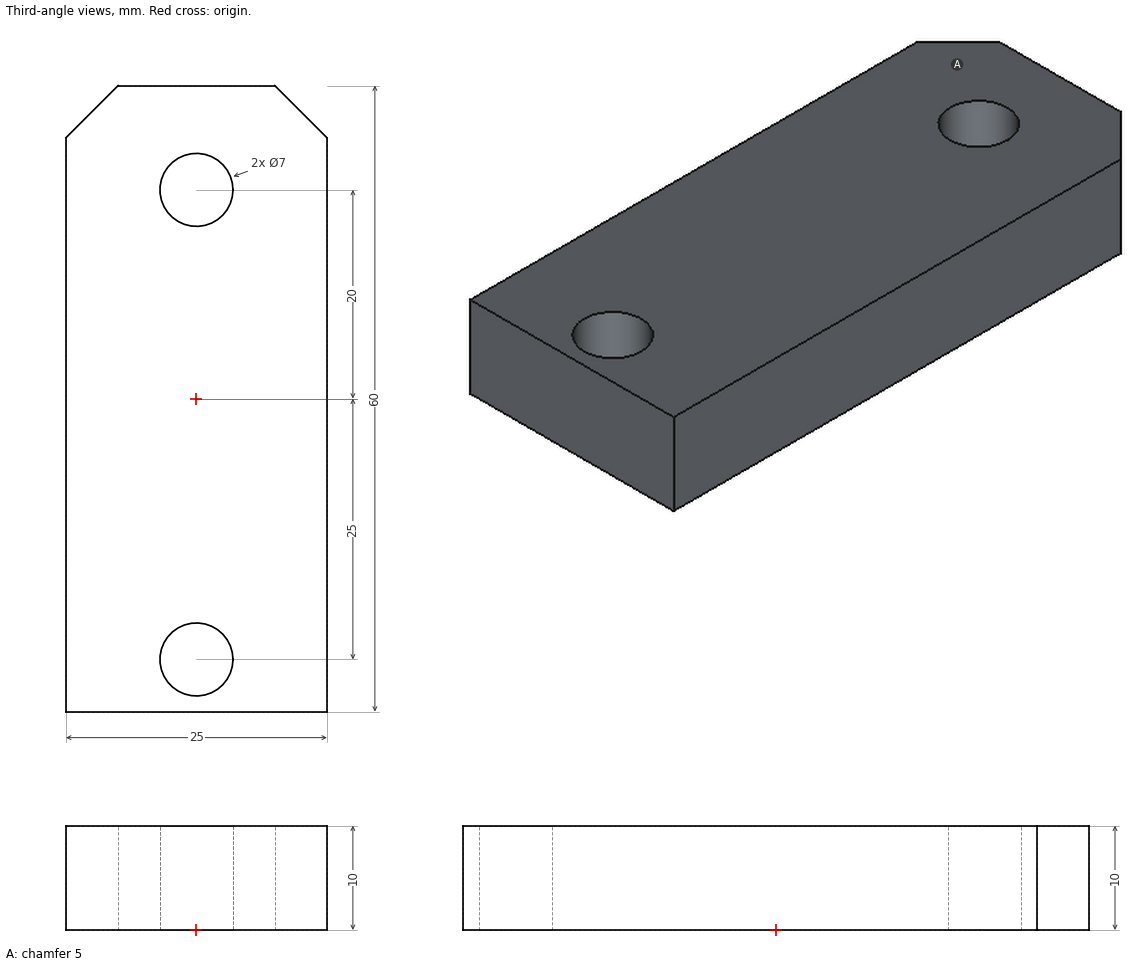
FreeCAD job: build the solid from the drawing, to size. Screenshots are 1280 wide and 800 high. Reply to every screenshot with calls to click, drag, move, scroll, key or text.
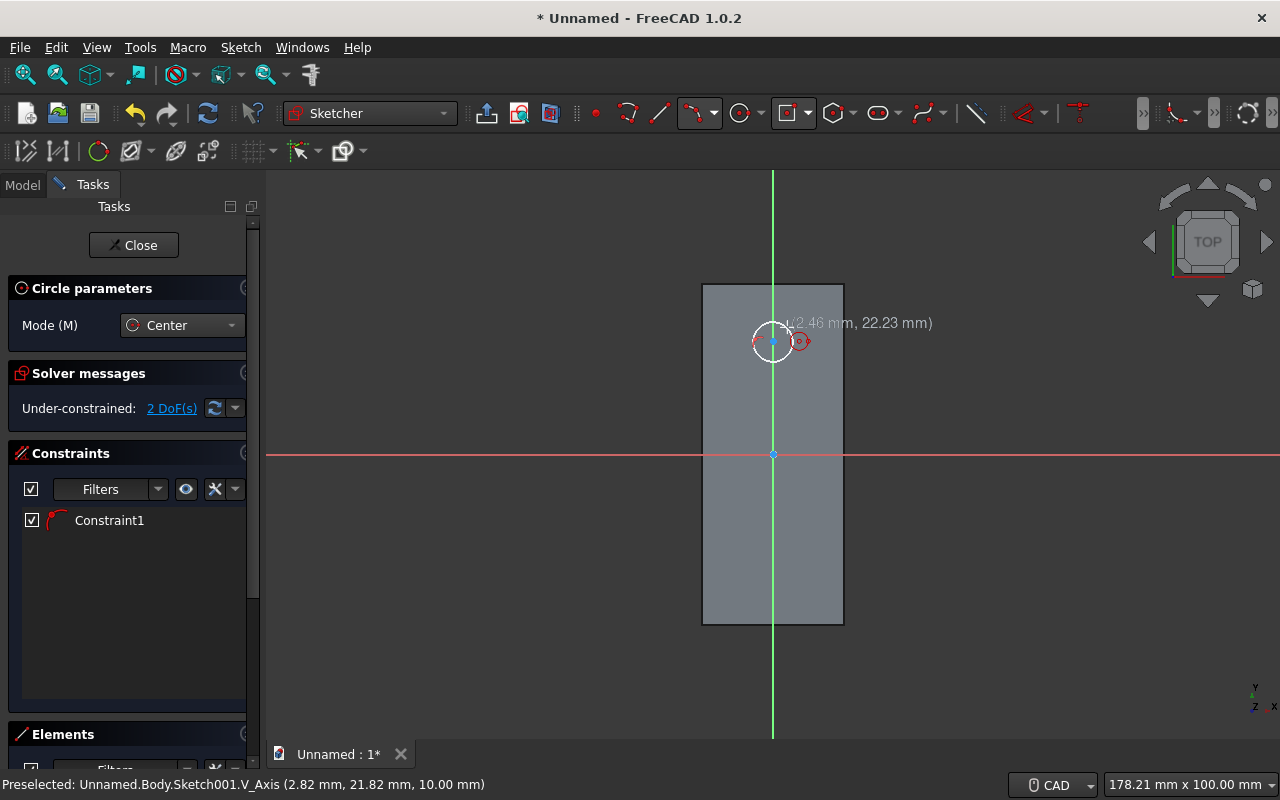
click(773, 597)
click(787, 583)
key(Escape)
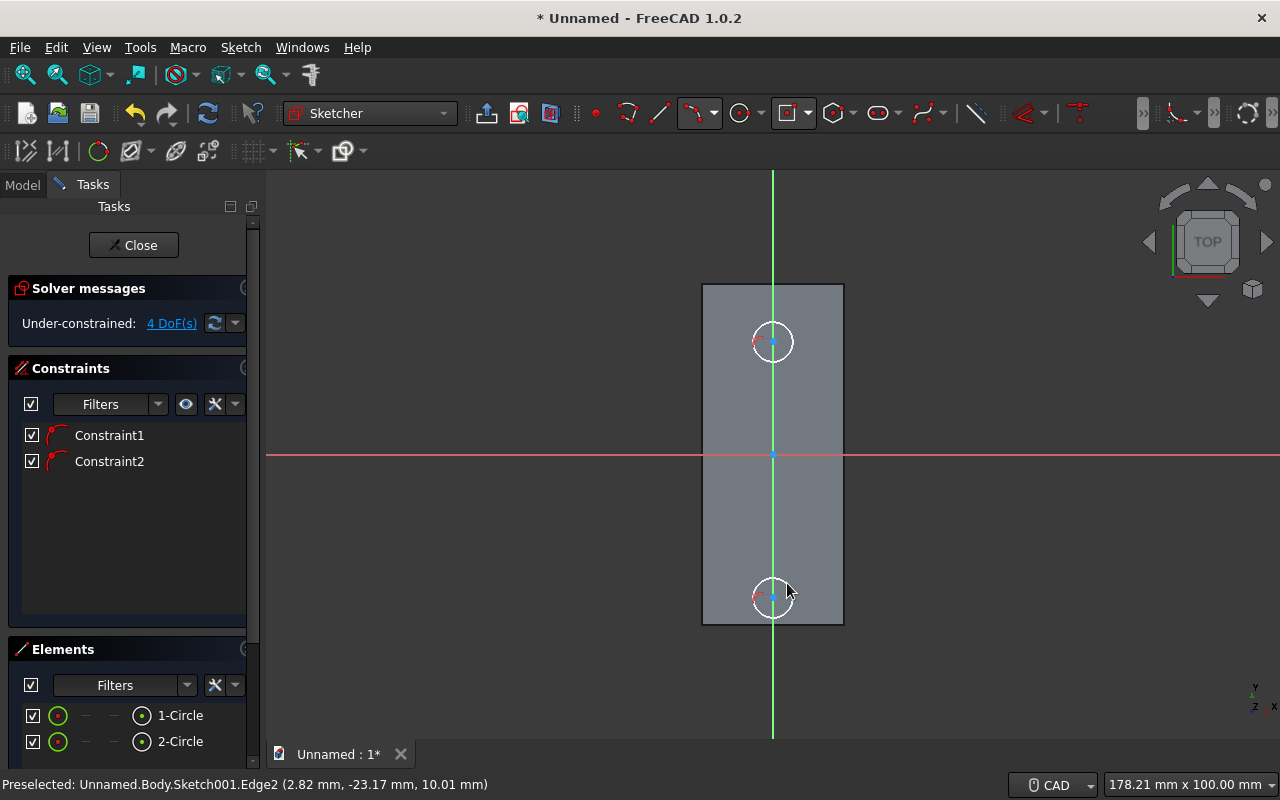
click(787, 328)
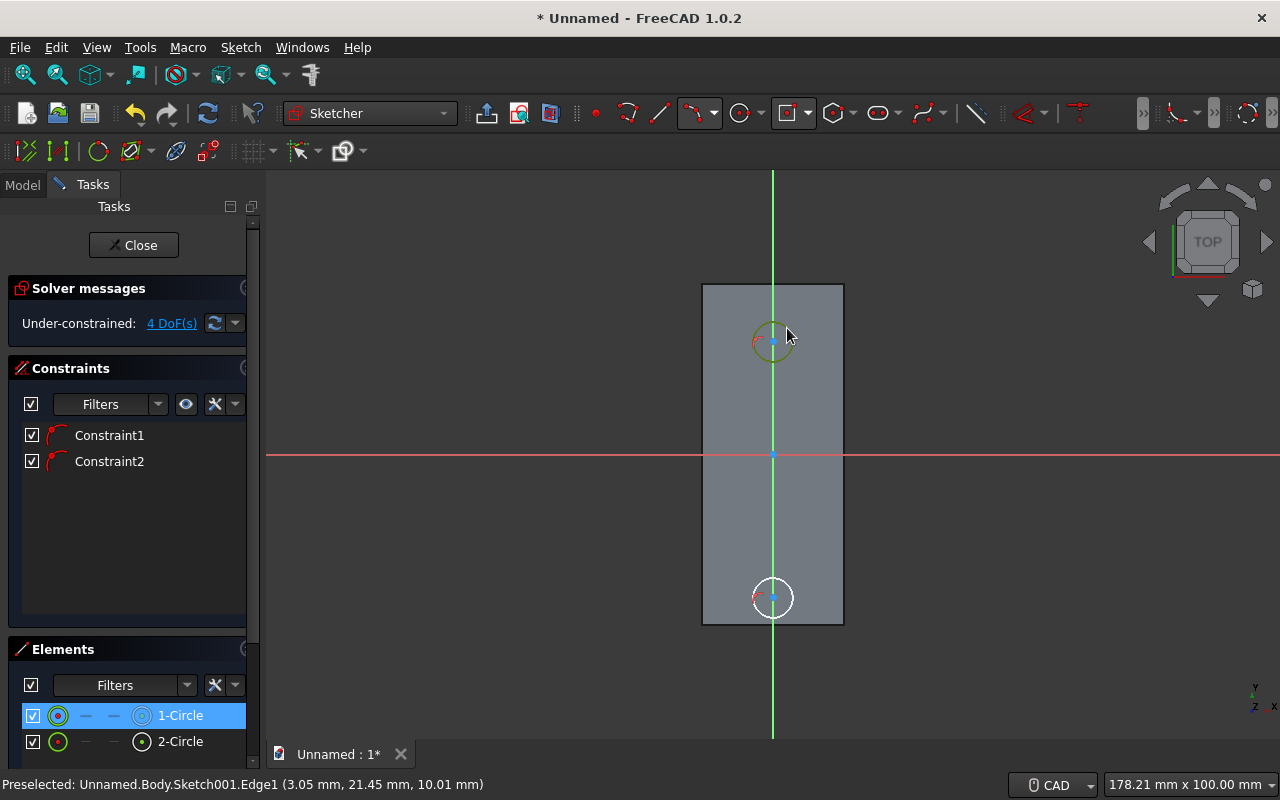
click(787, 584)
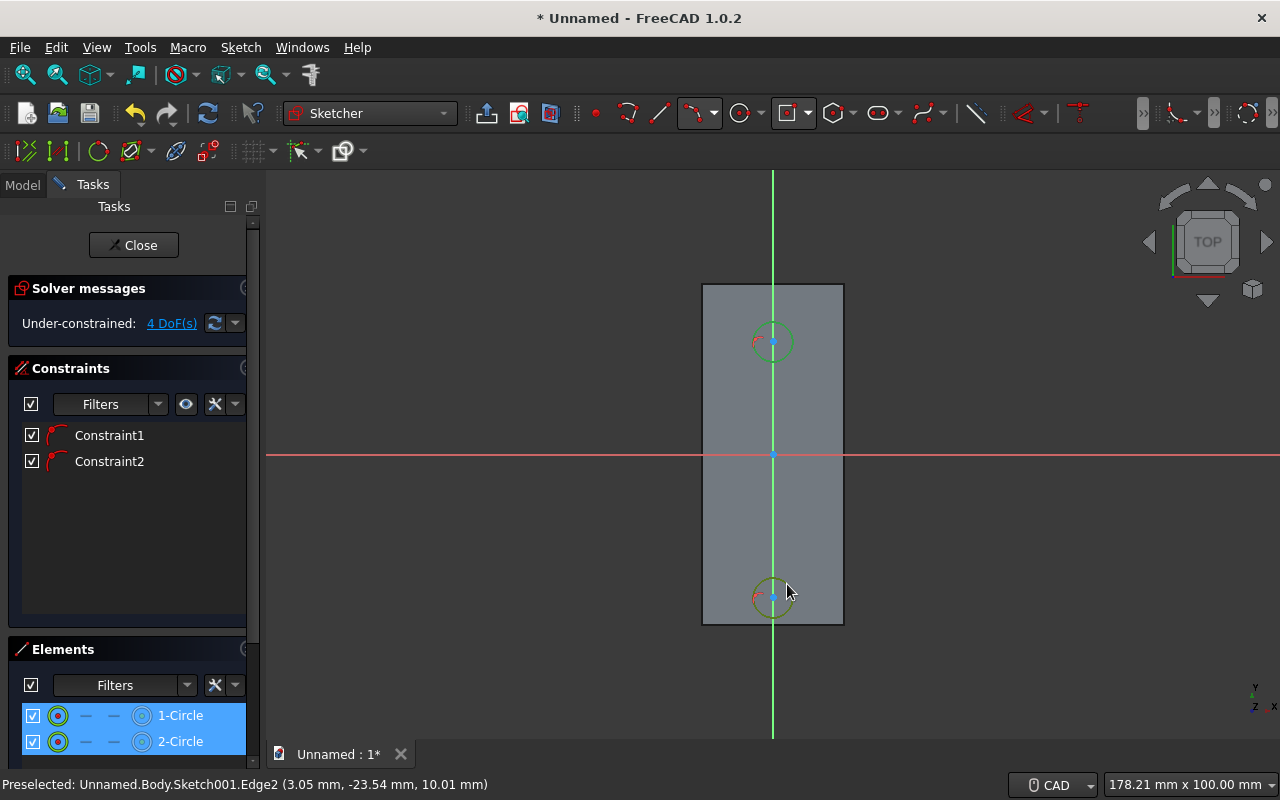
key(e)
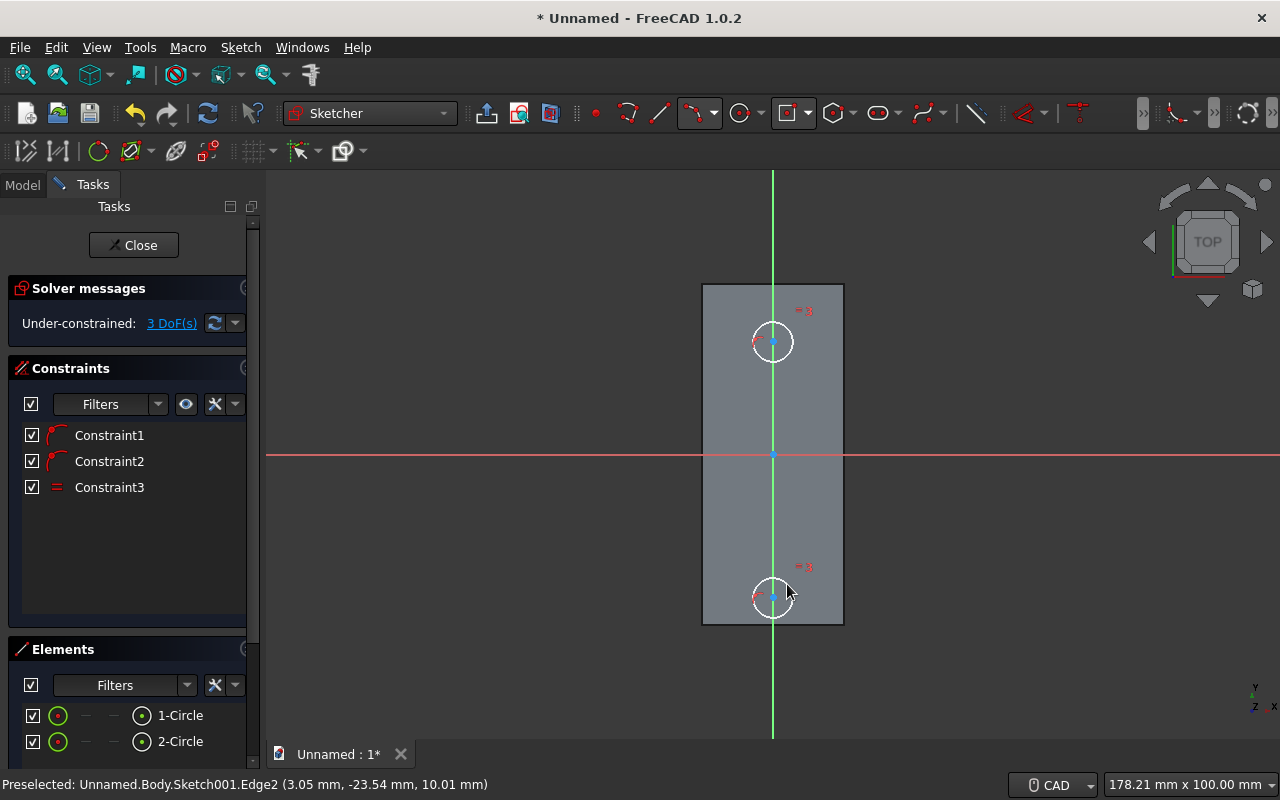
click(1024, 114)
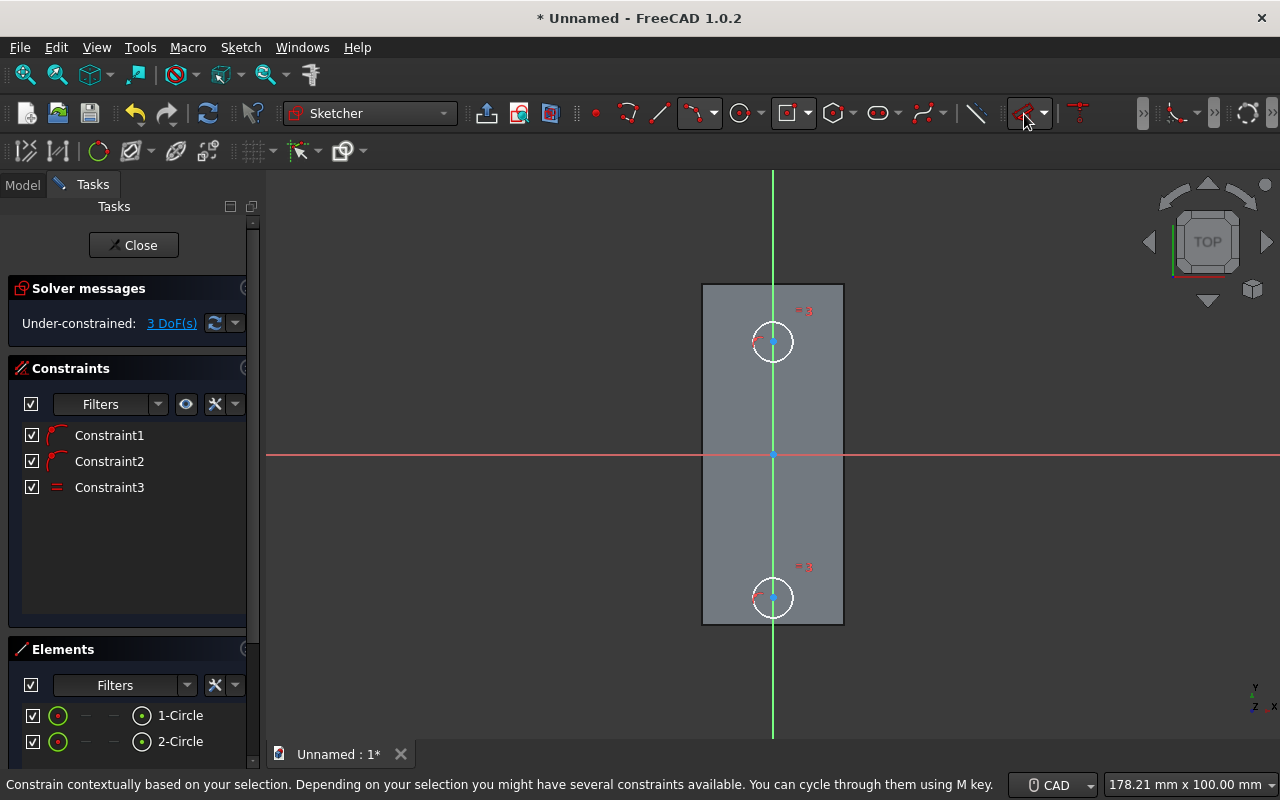
click(787, 328)
click(810, 305)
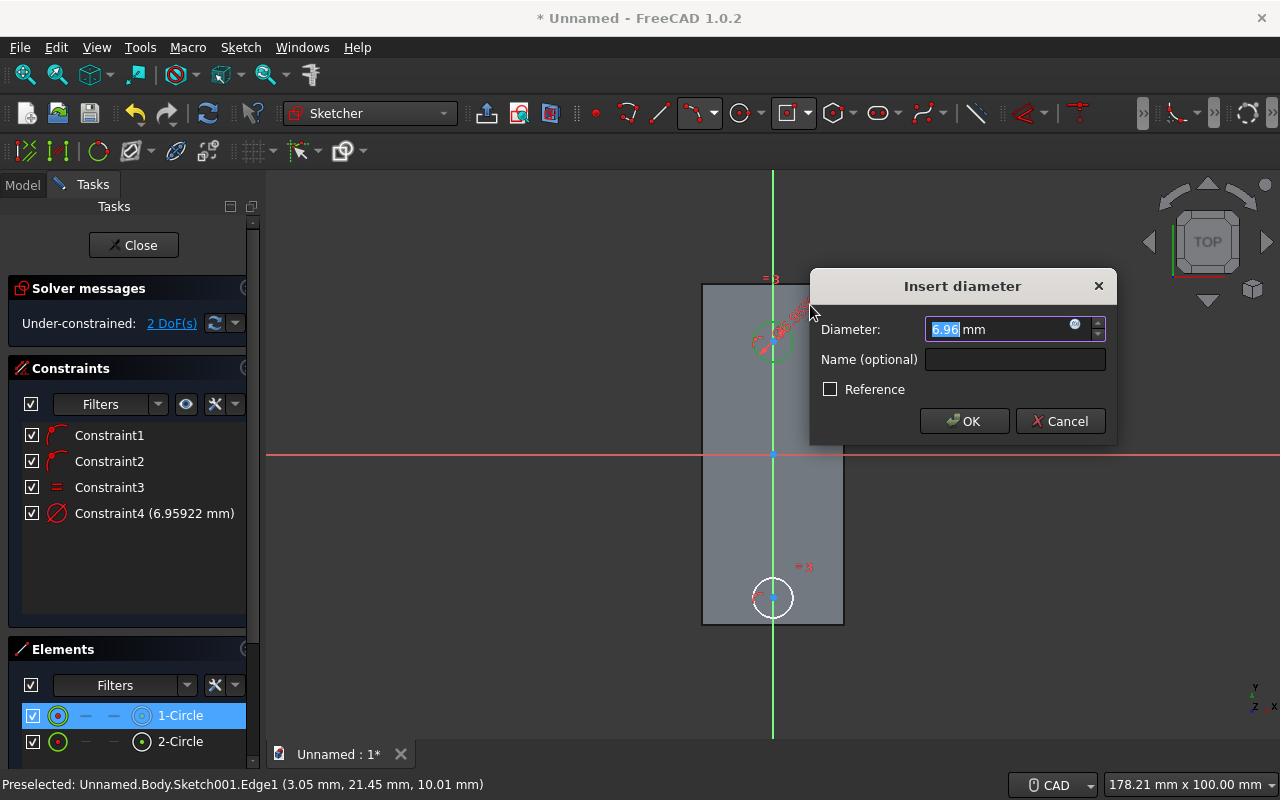
text(7)
key(Return)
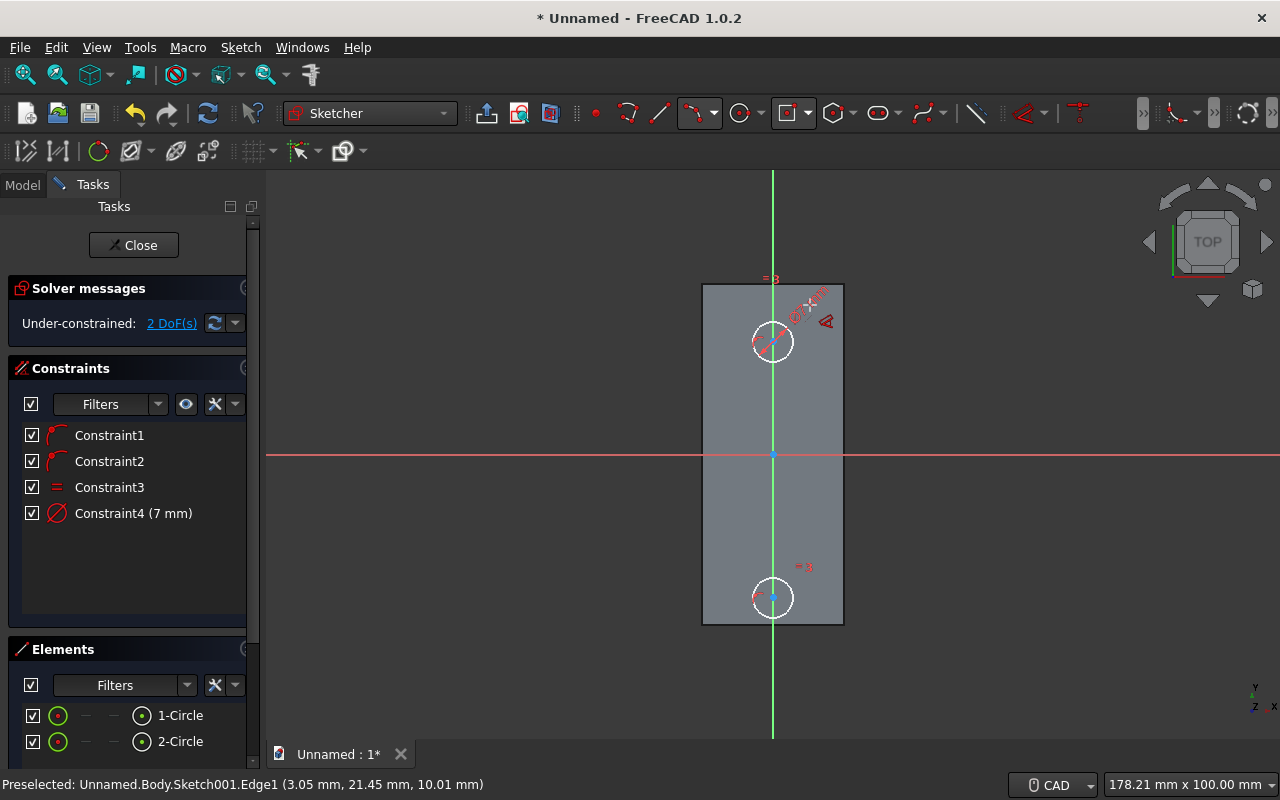
click(773, 342)
click(807, 398)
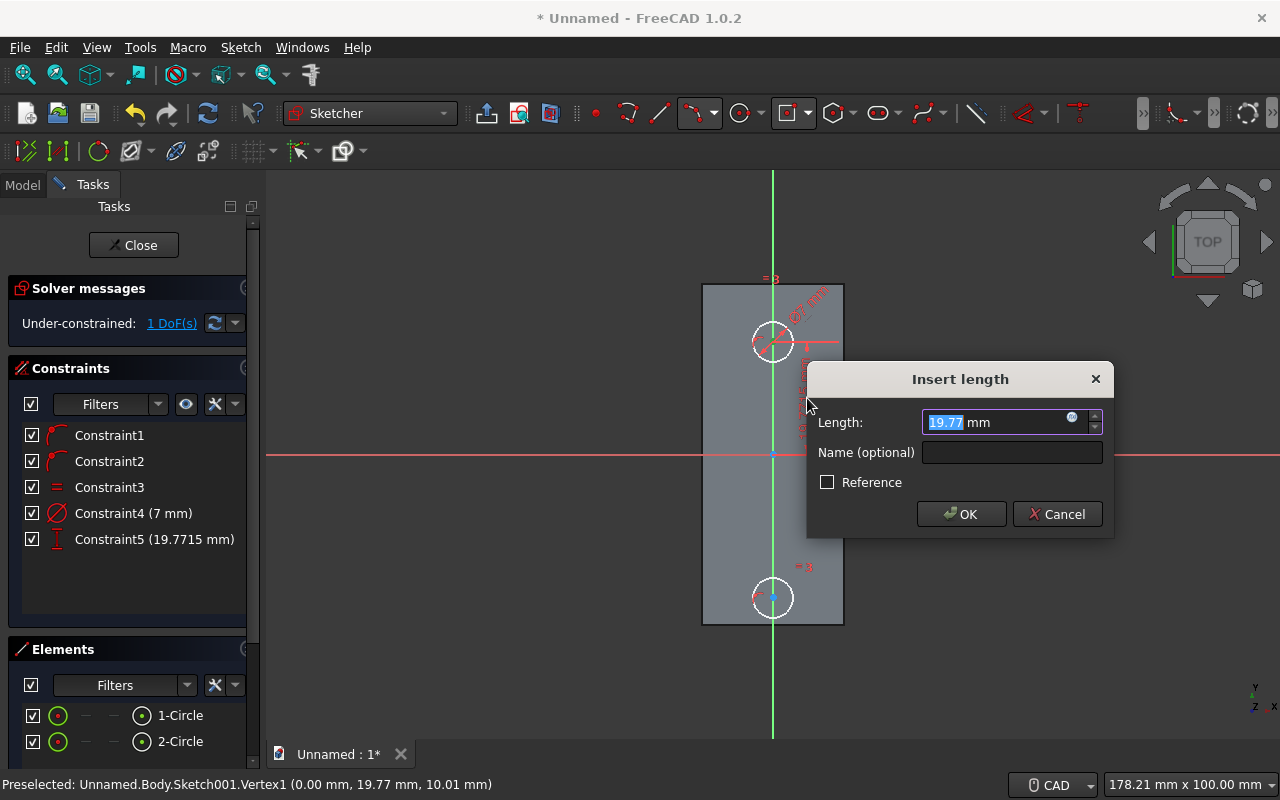
text(20)
key(Return)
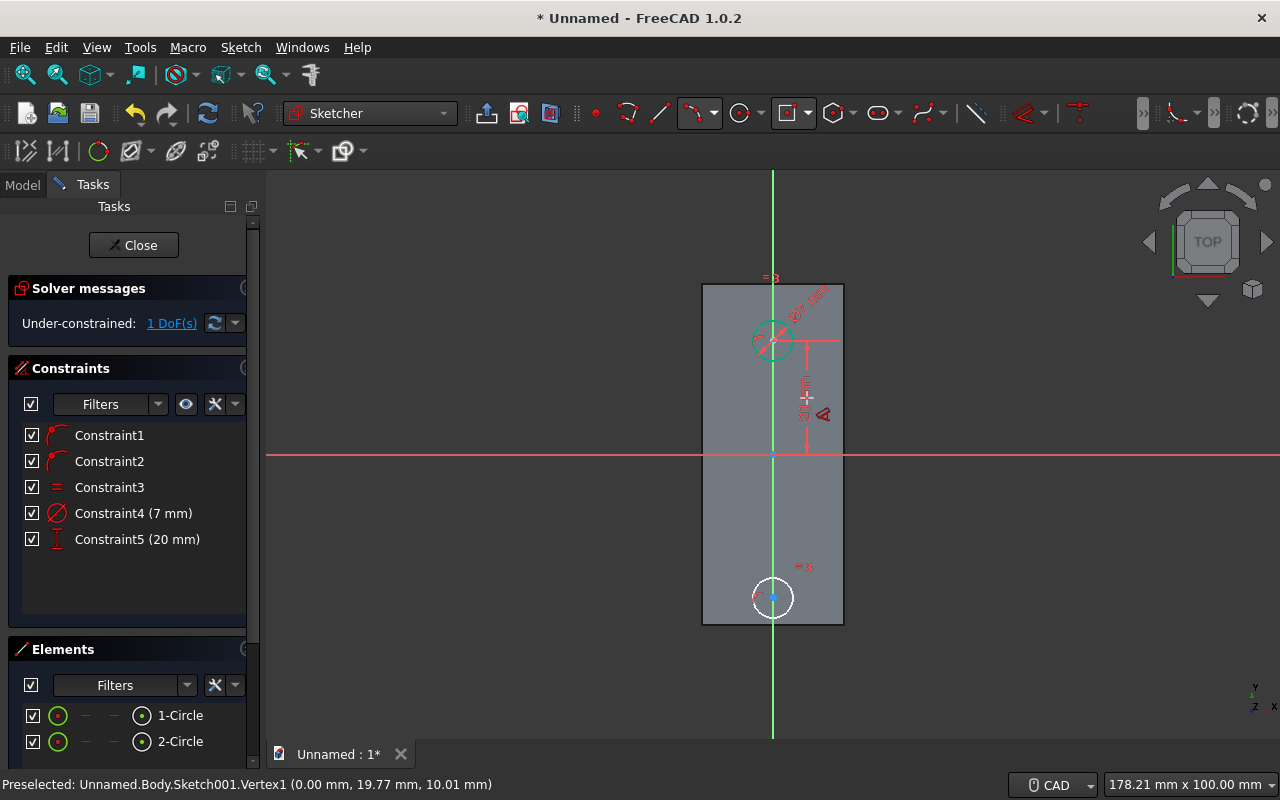
click(773, 598)
click(807, 526)